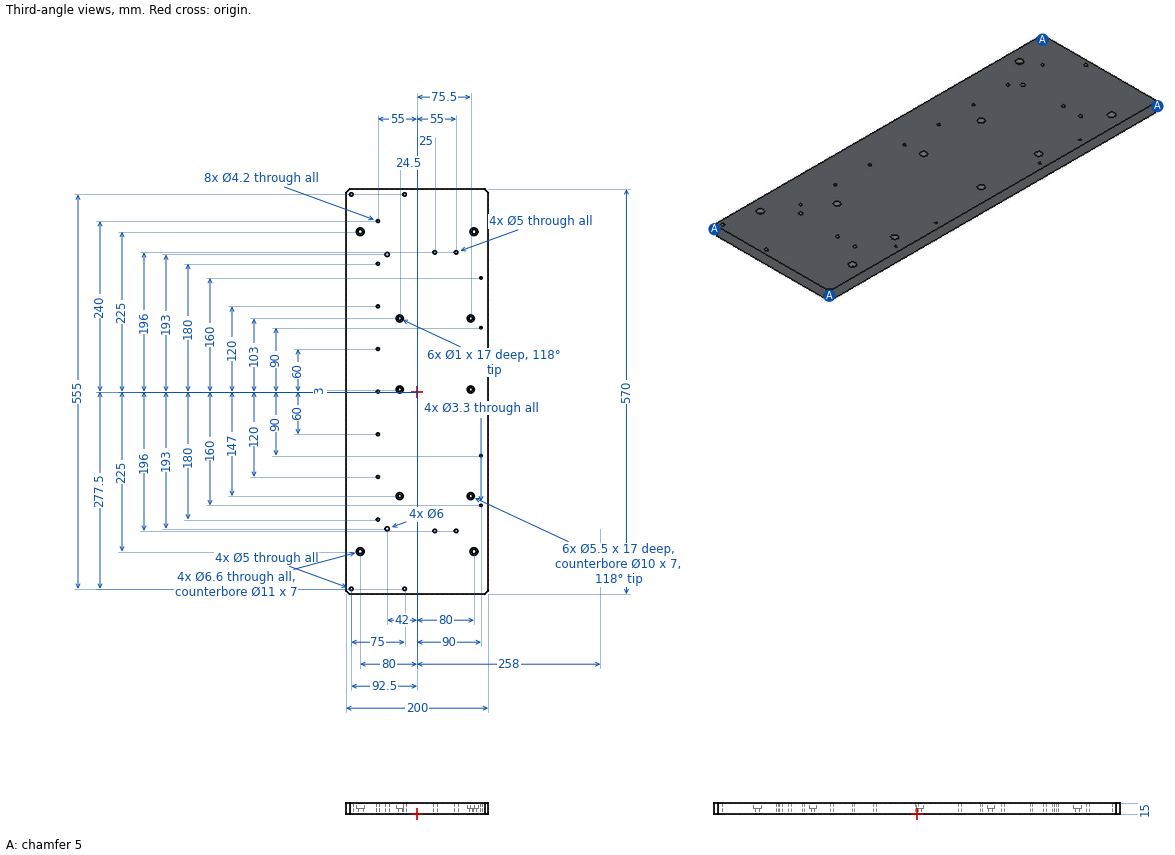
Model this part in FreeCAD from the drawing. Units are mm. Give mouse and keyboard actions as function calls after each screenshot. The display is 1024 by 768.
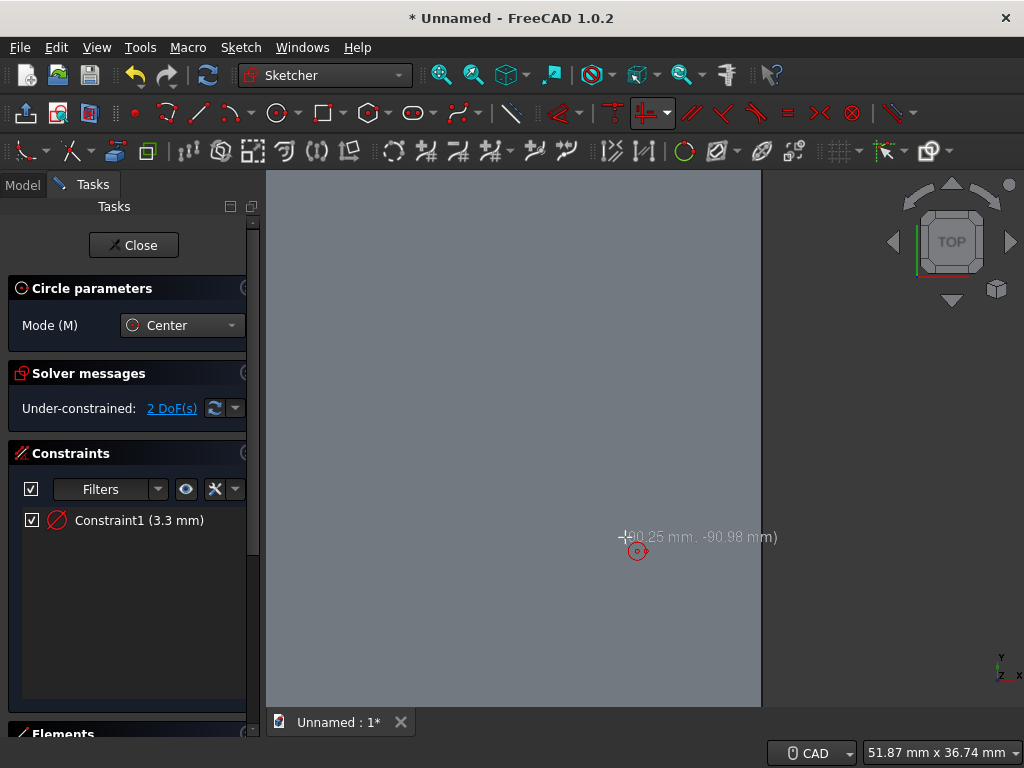
scroll(625, 537, down, 13)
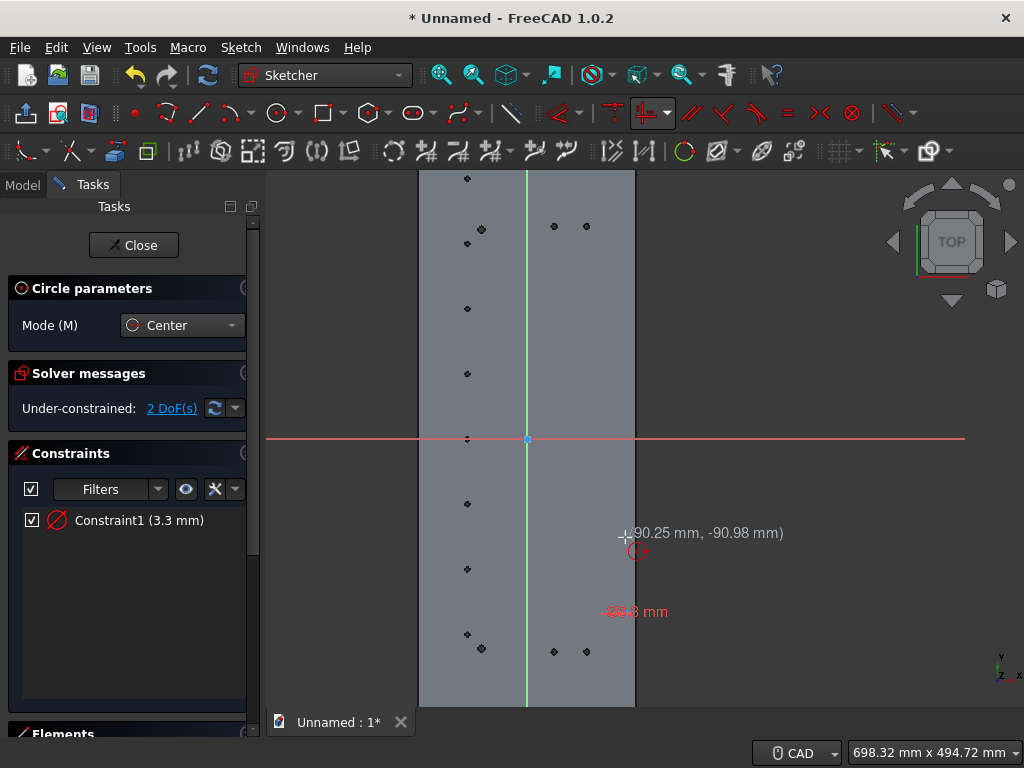
click(625, 537)
move(626, 536)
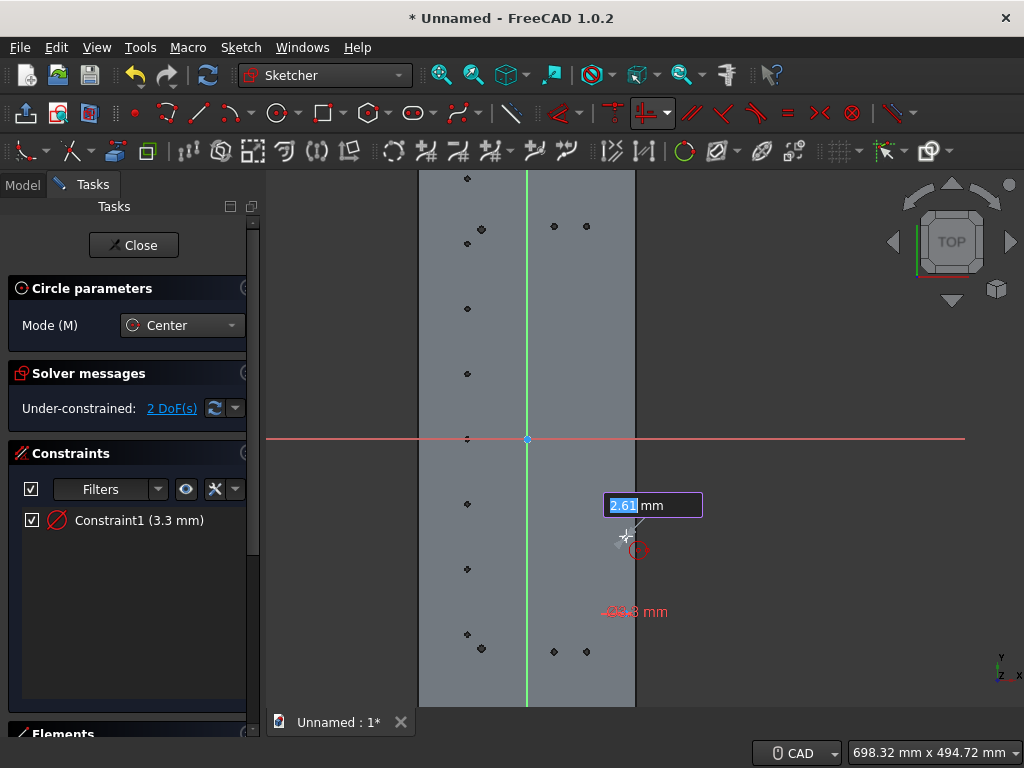
text(3.3)
key(Return)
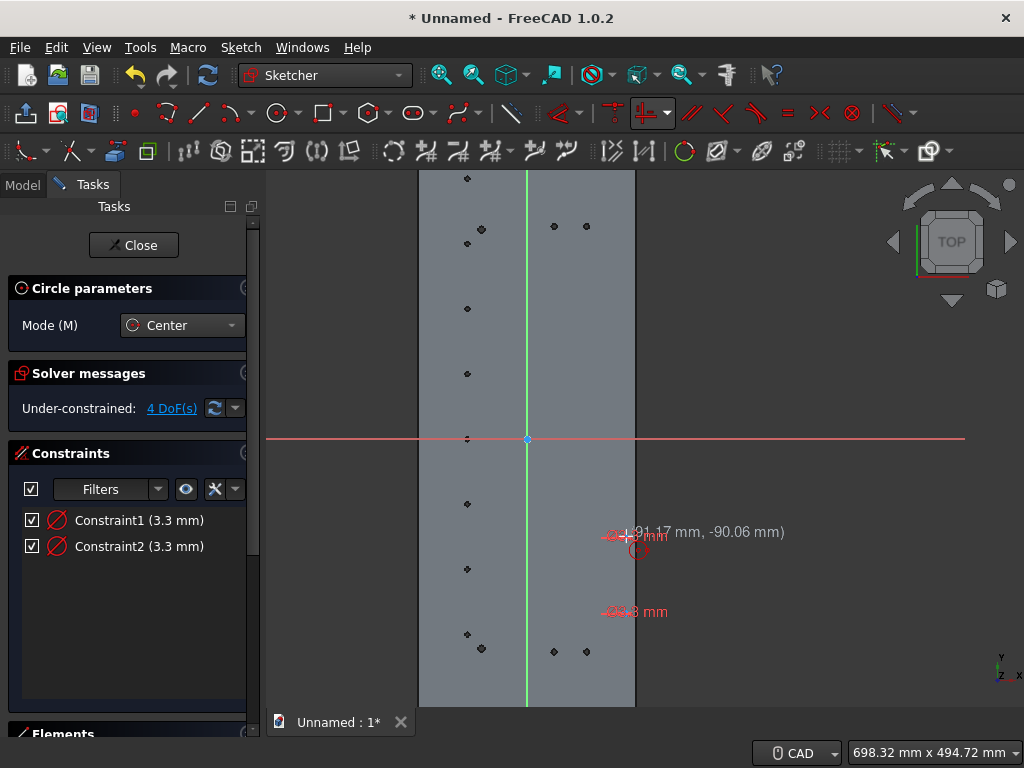
scroll(625, 342, up, 13)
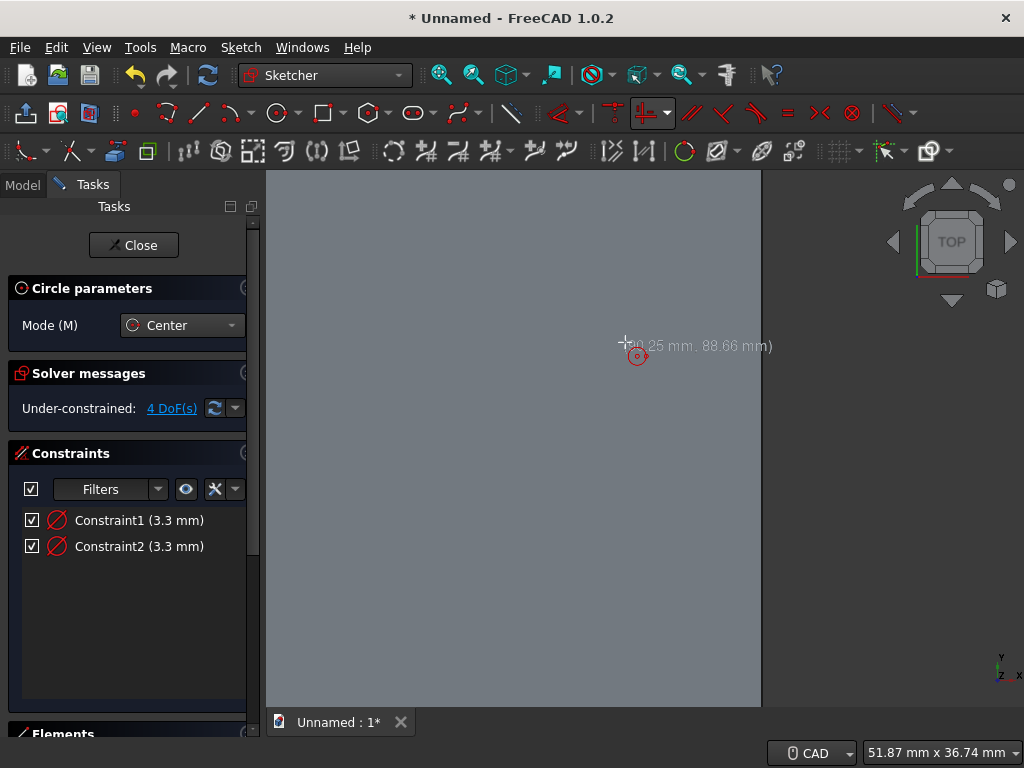
scroll(625, 342, down, 13)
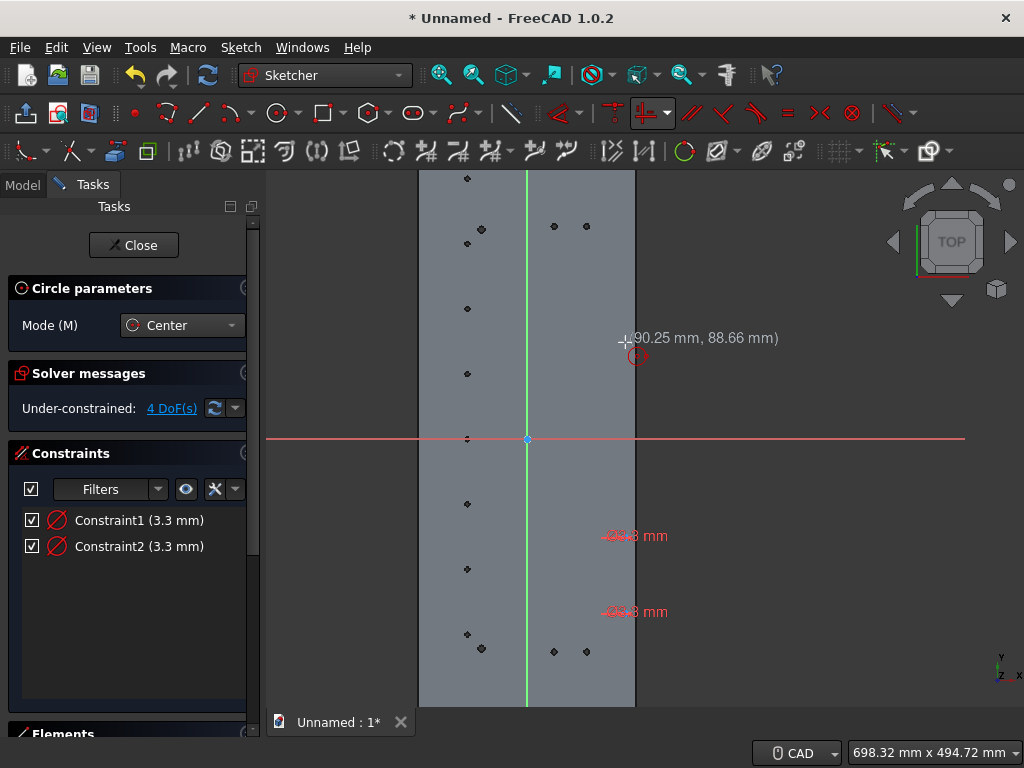
click(625, 342)
move(626, 340)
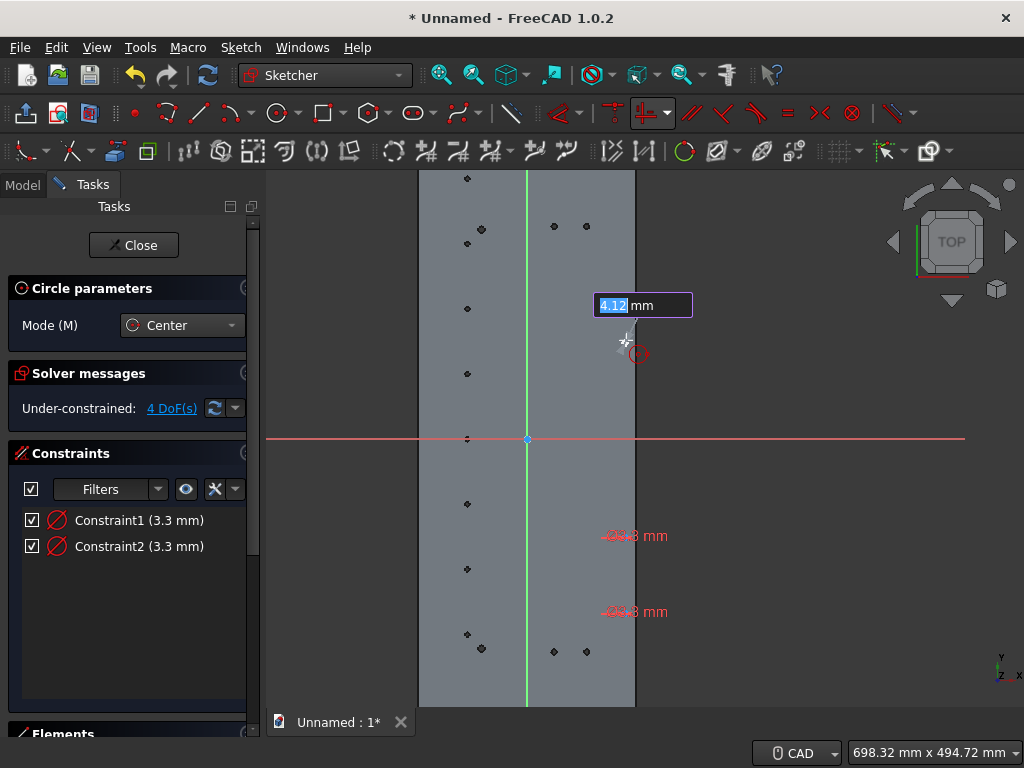
text(3.3)
key(Return)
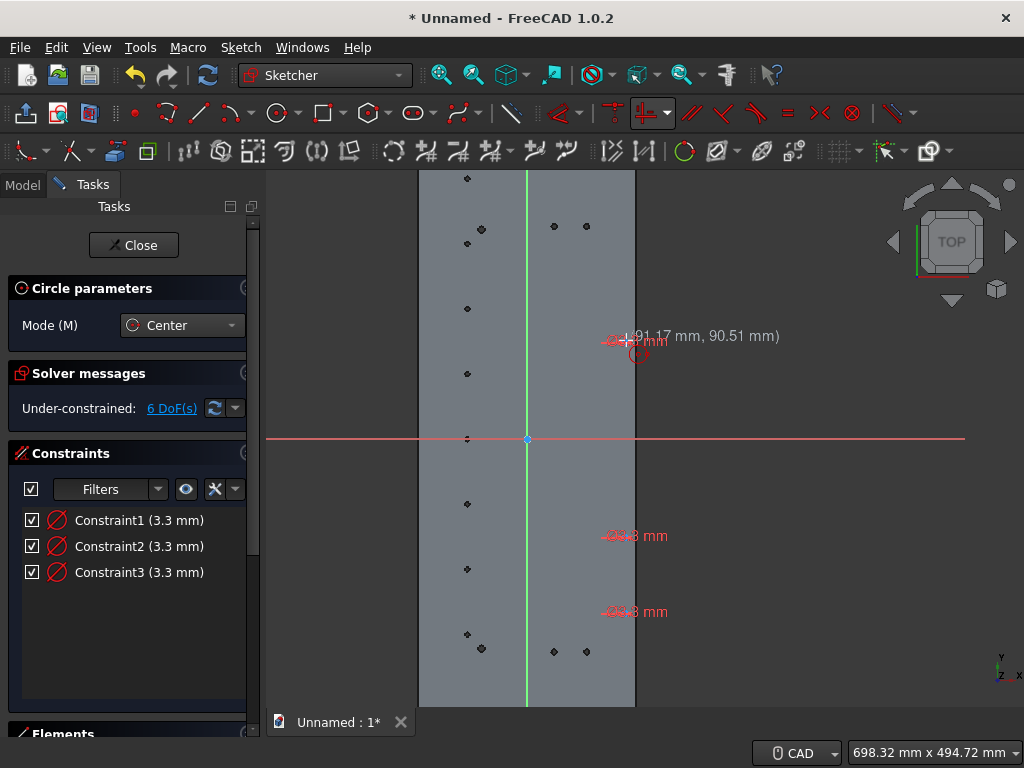
scroll(625, 266, up, 13)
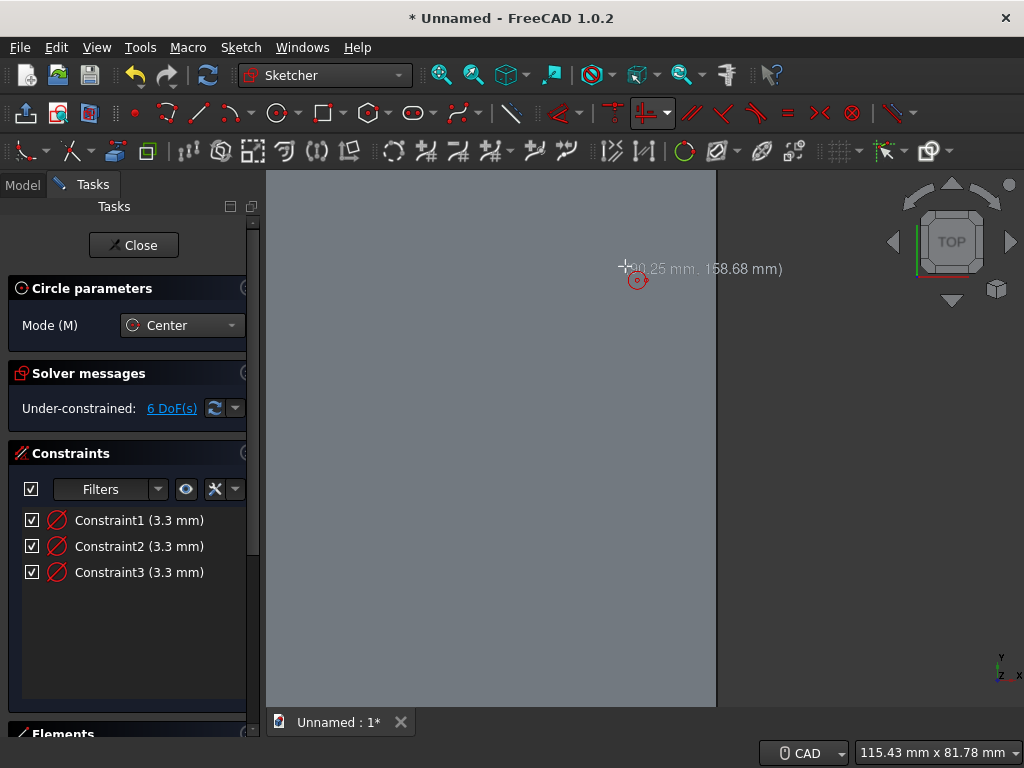
scroll(625, 265, down, 13)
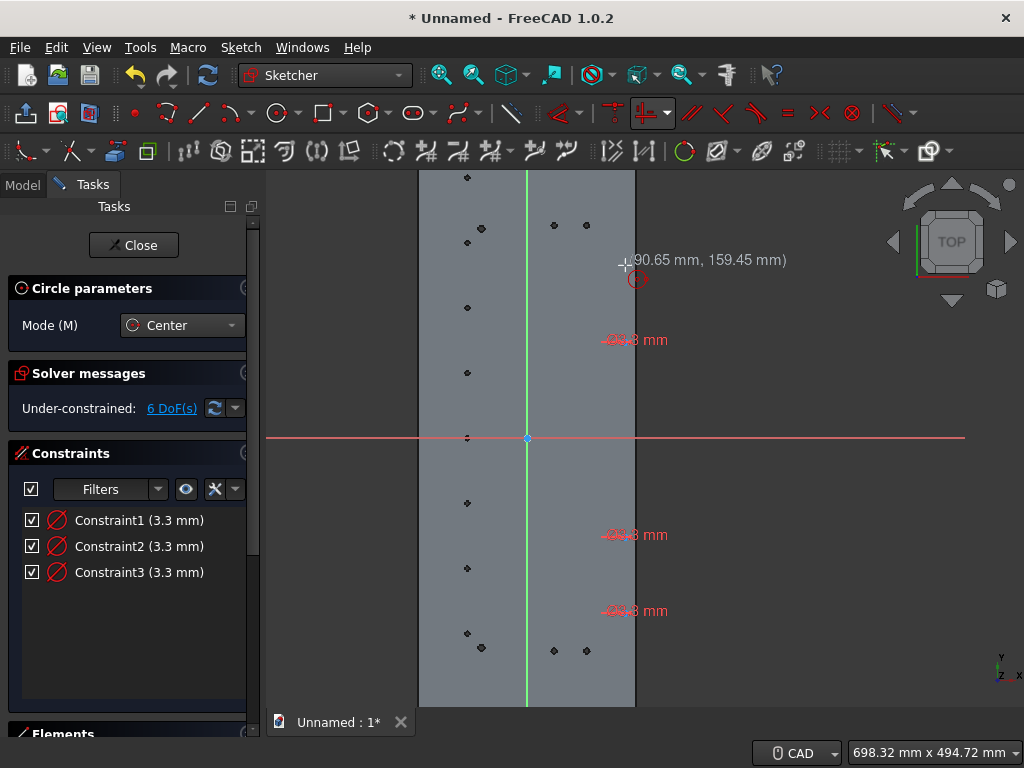
click(625, 265)
move(626, 263)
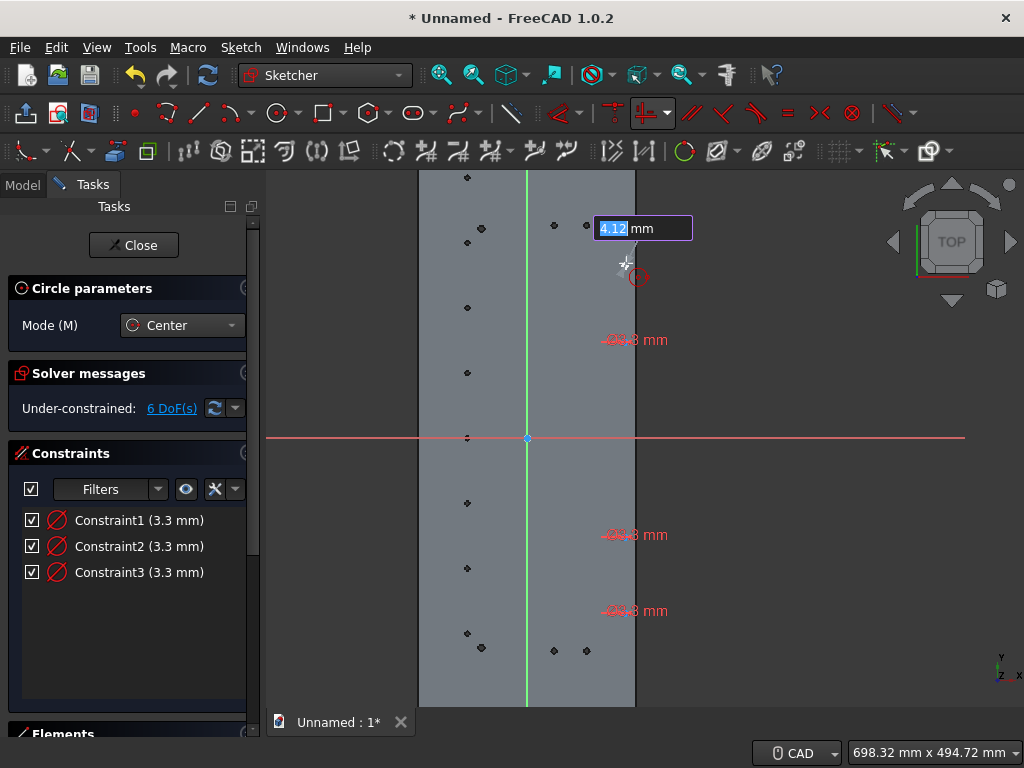
text(3.3)
key(Return)
key(Escape)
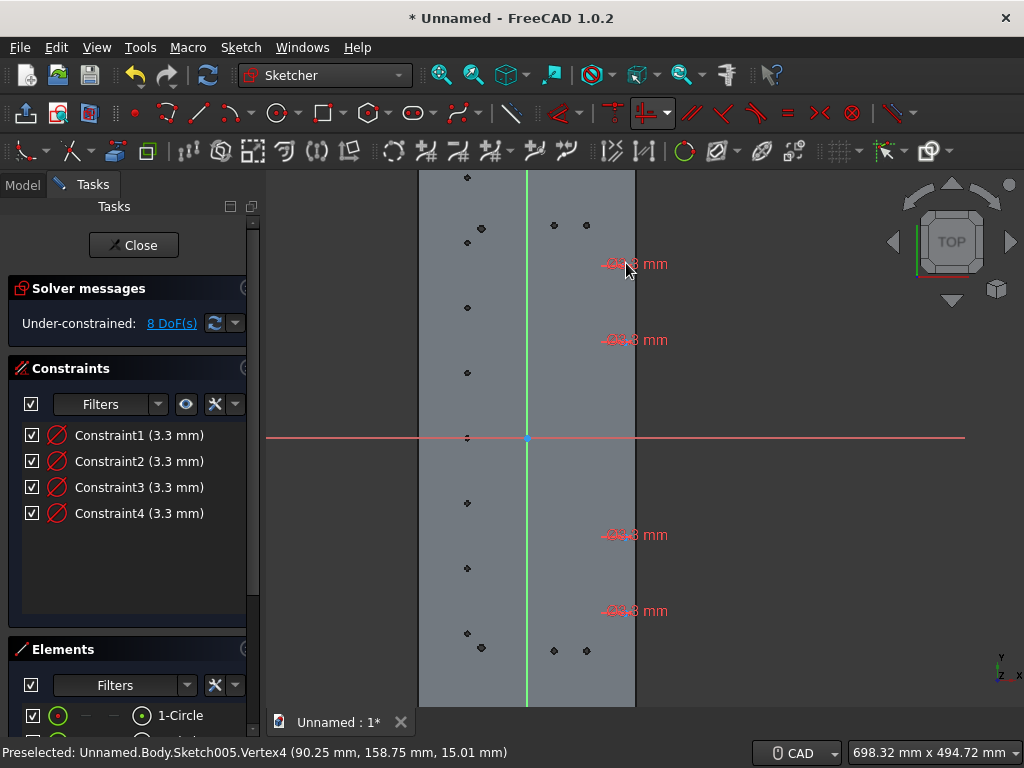
click(625, 613)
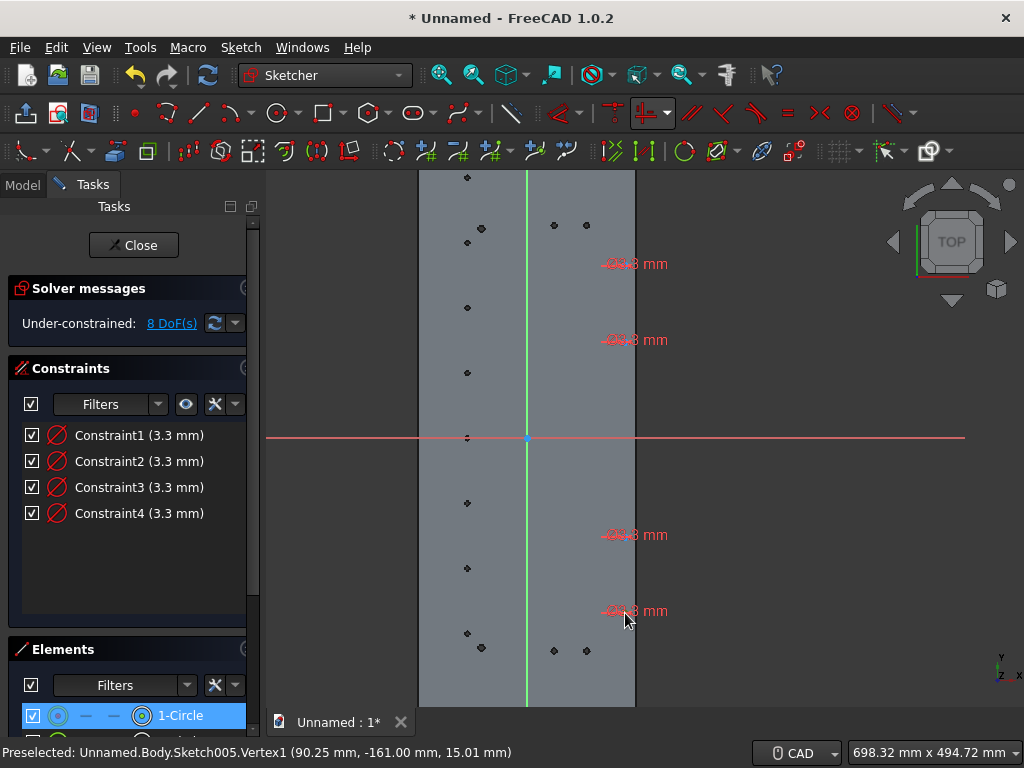
click(625, 537)